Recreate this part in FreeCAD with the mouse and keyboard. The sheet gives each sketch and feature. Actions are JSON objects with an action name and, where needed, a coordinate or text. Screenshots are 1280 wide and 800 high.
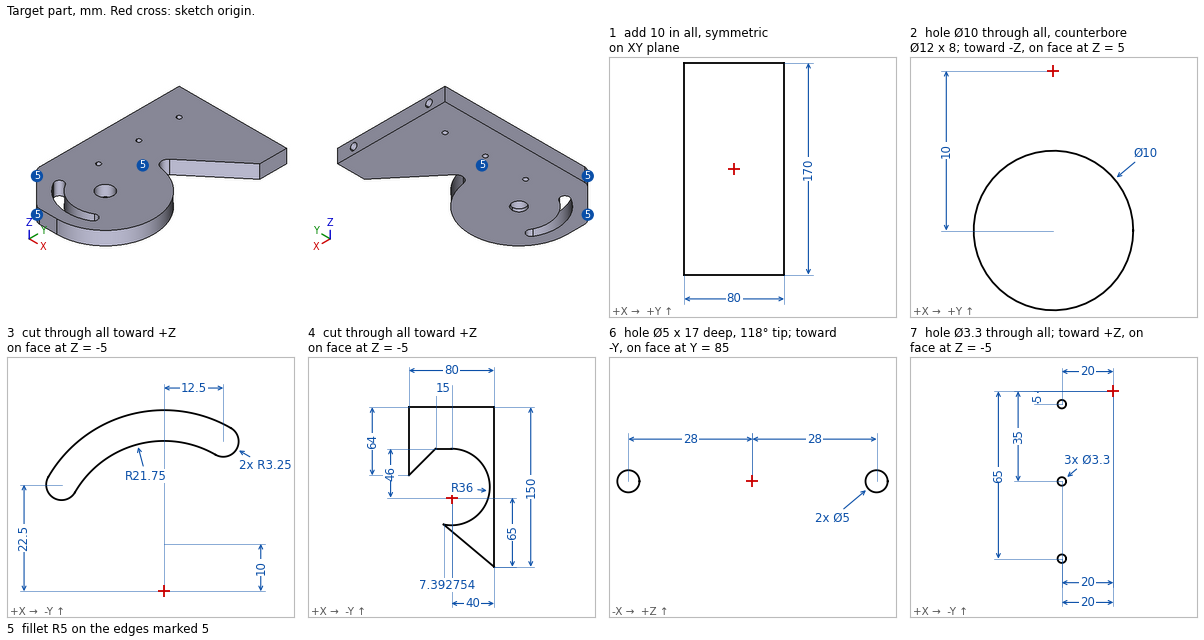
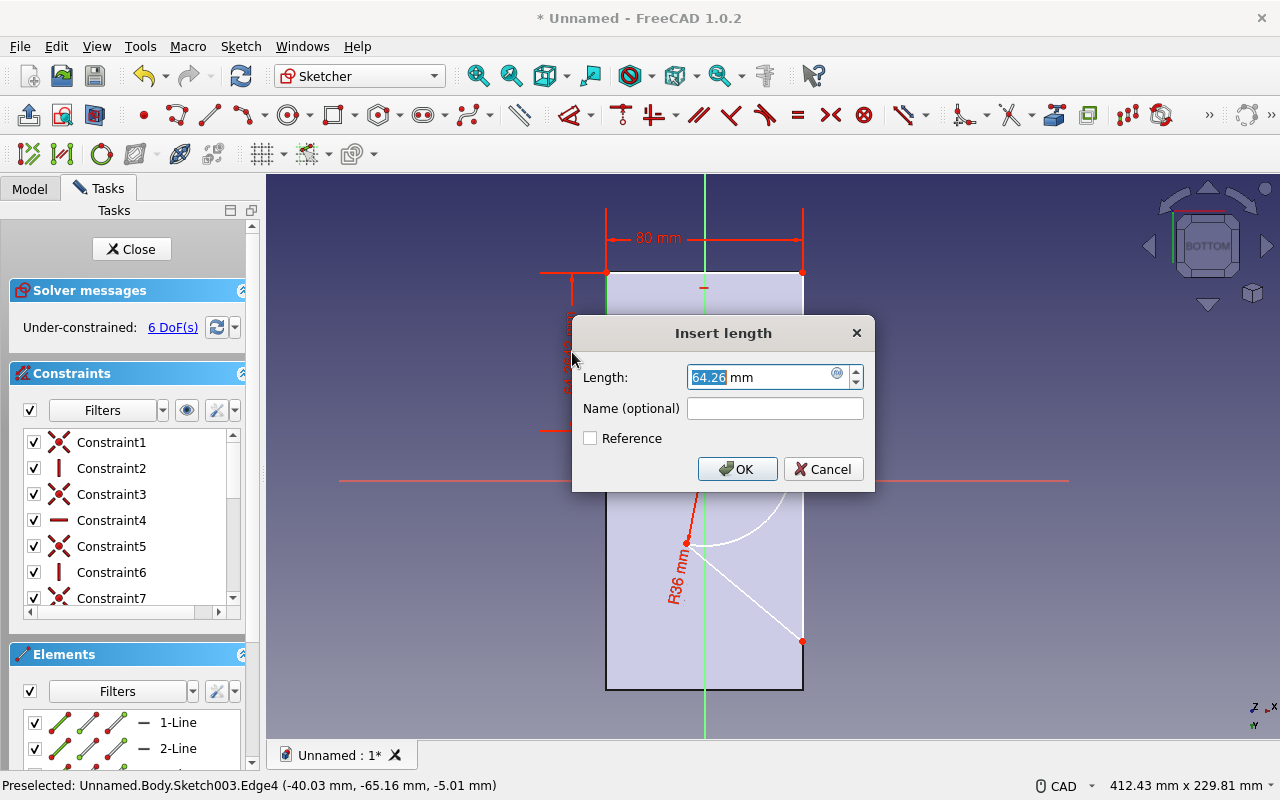
{"action": "type", "text": "64"}
{"action": "key", "text": "Return"}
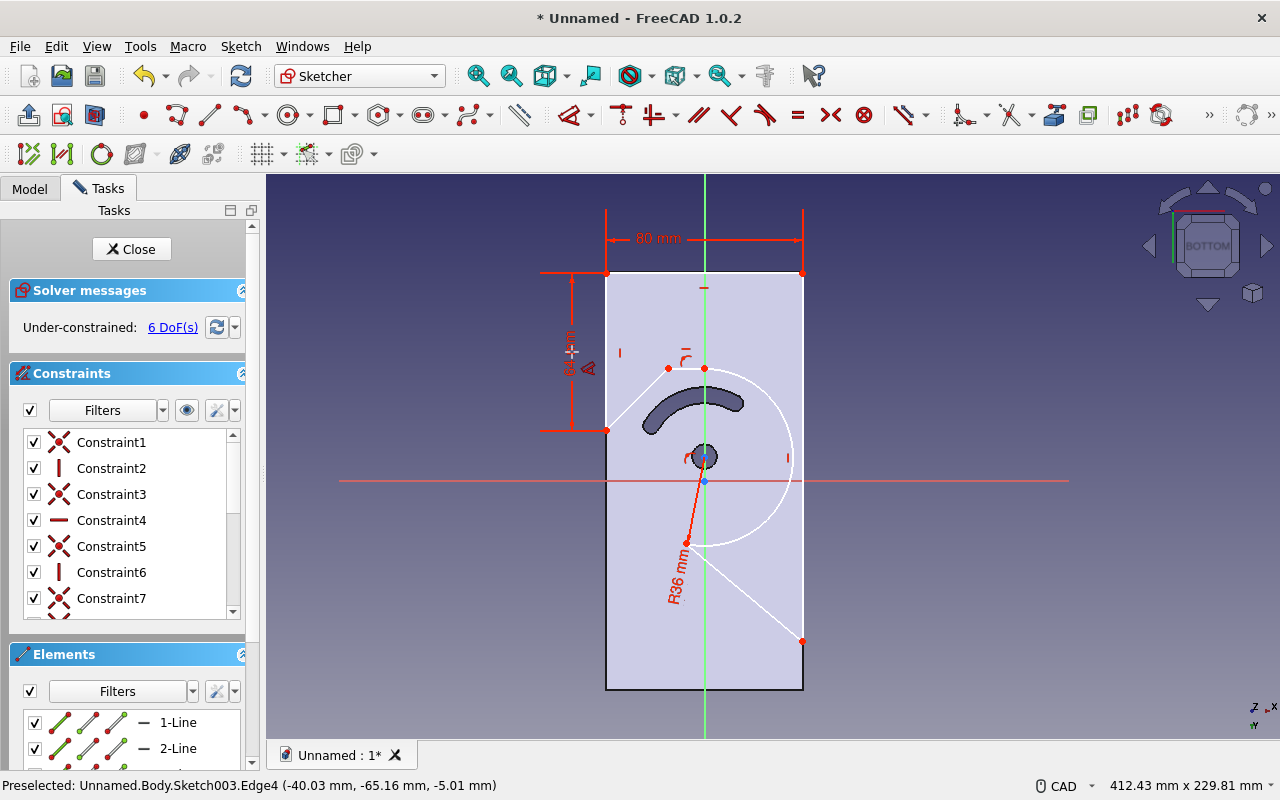
{"action": "scroll", "coordinate": [679, 369], "scroll_direction": "up", "scroll_amount": 2}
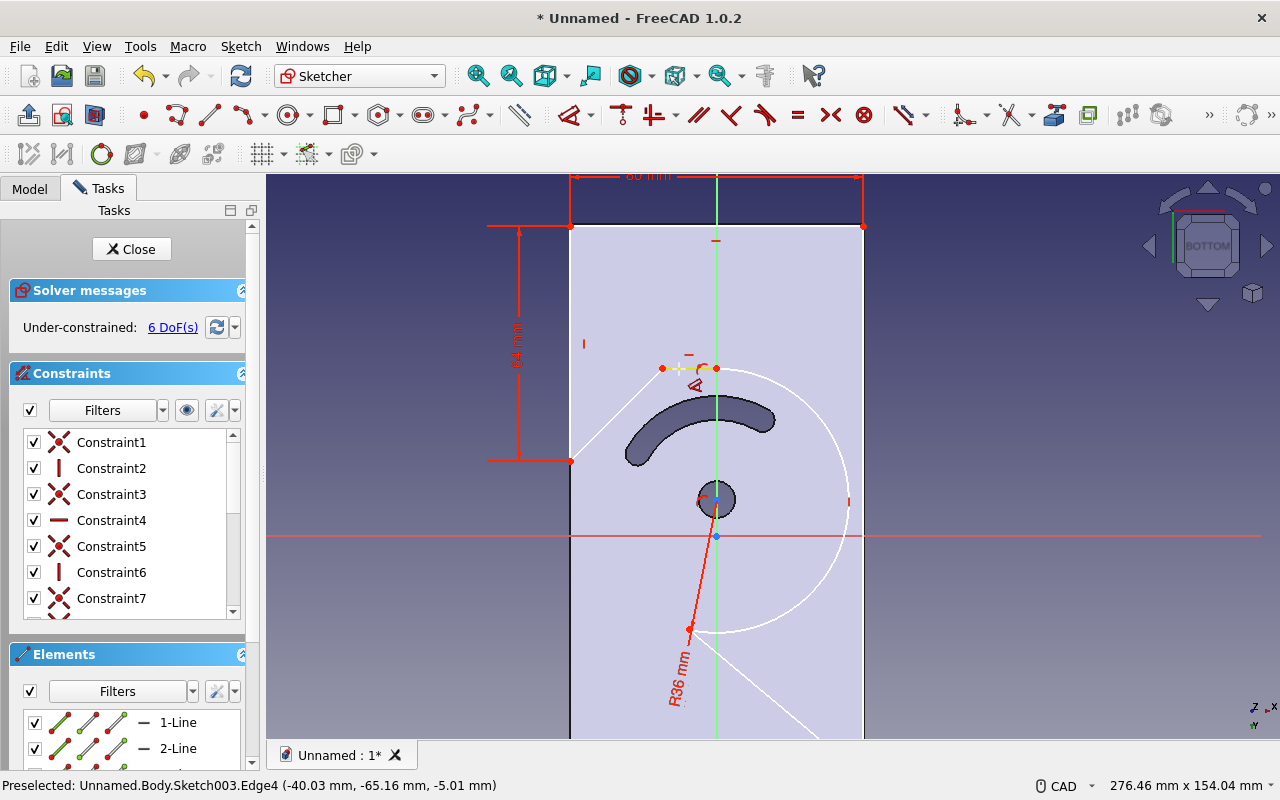
{"action": "left_click", "coordinate": [679, 369]}
{"action": "left_click", "coordinate": [690, 335]}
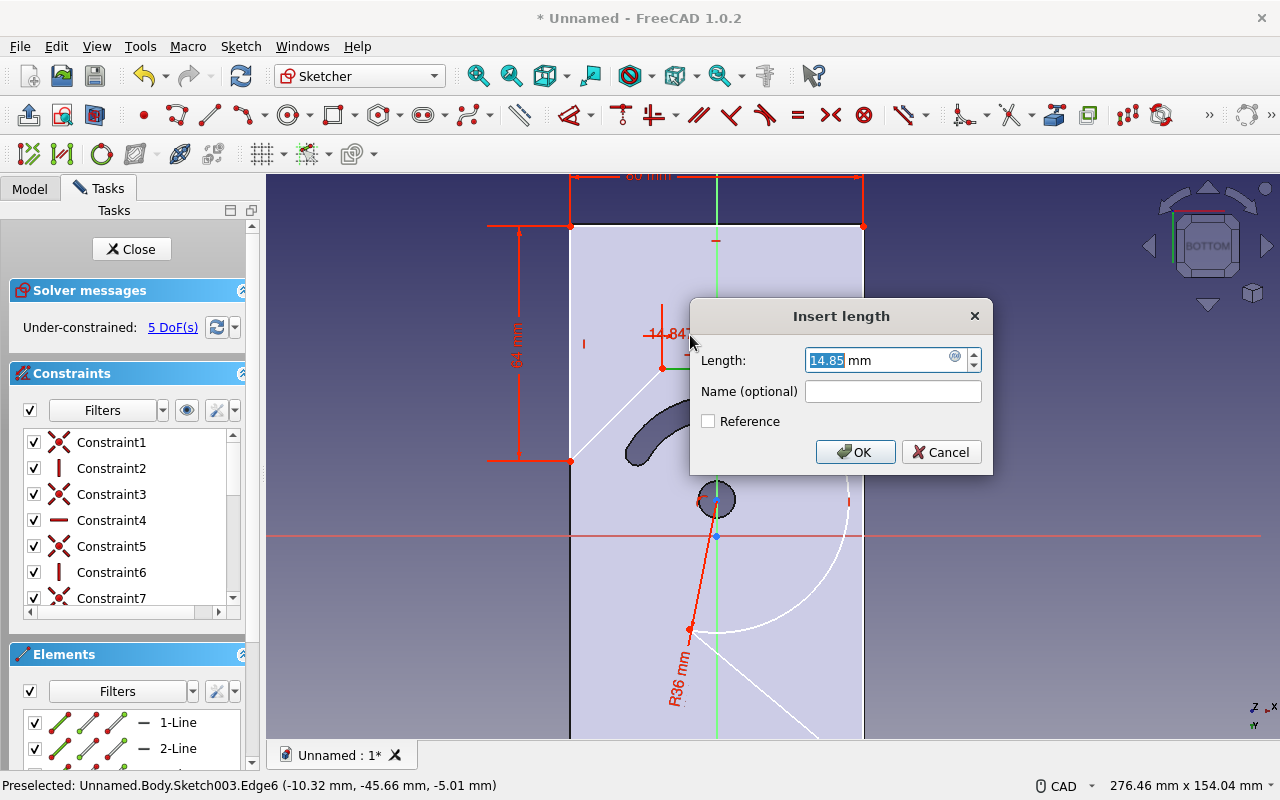
{"action": "type", "text": "15"}
{"action": "key", "text": "Return"}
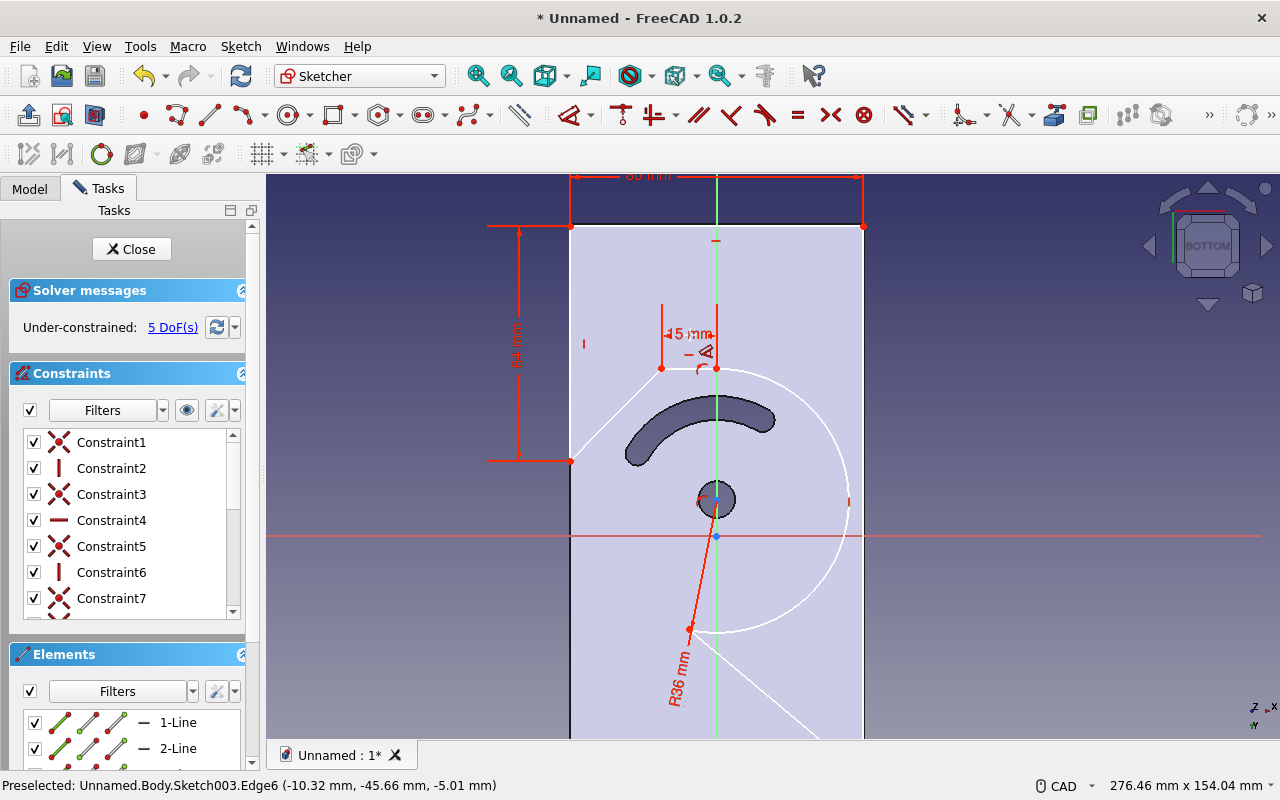
{"action": "left_click", "coordinate": [863, 611]}
{"action": "left_click", "coordinate": [897, 469]}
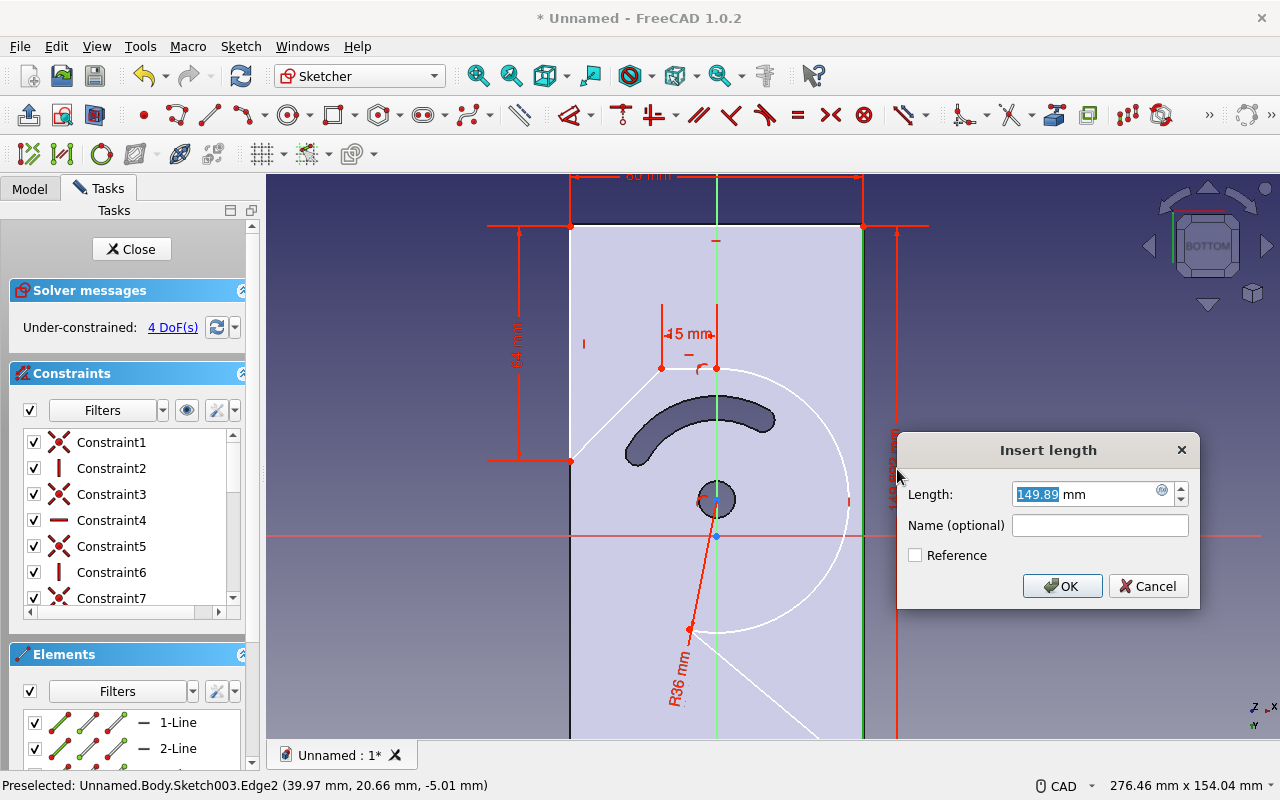
{"action": "type", "text": "150"}
{"action": "key", "text": "Return"}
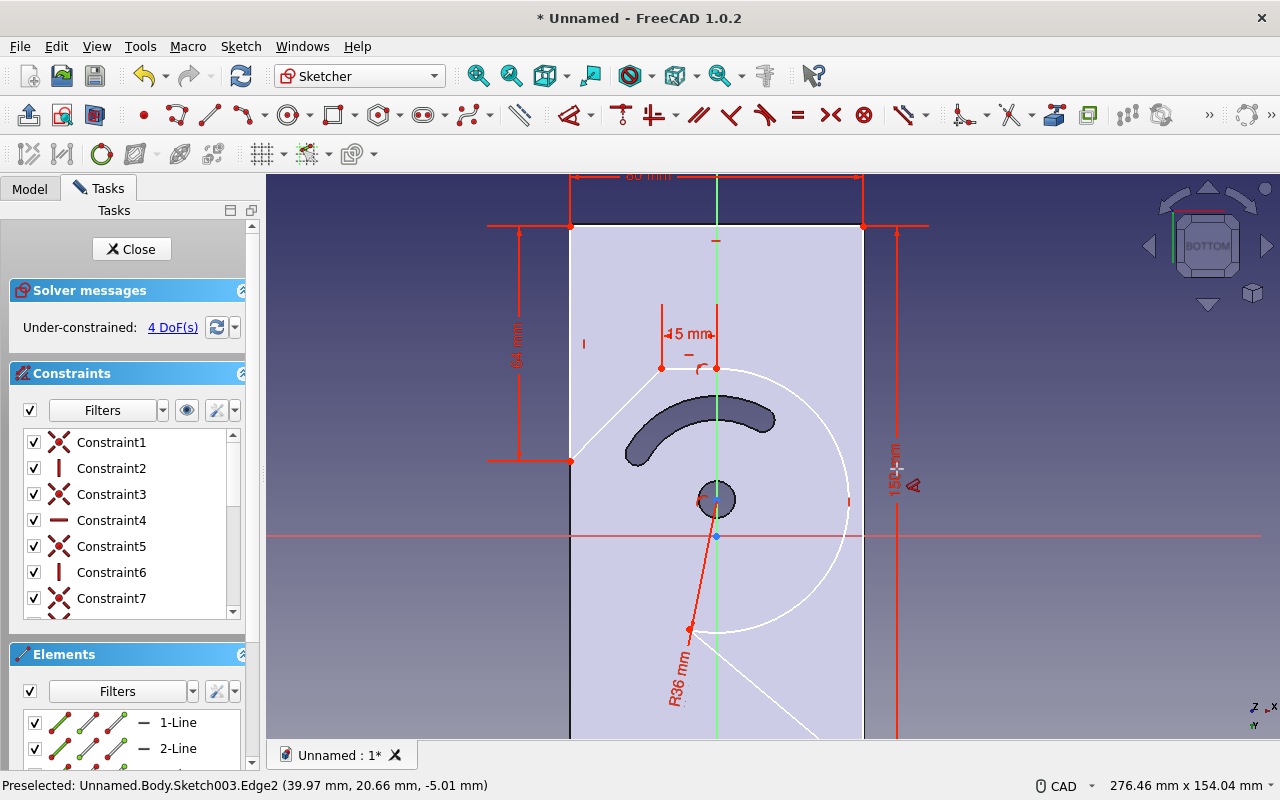
{"action": "scroll", "coordinate": [679, 369], "scroll_direction": "down", "scroll_amount": 2}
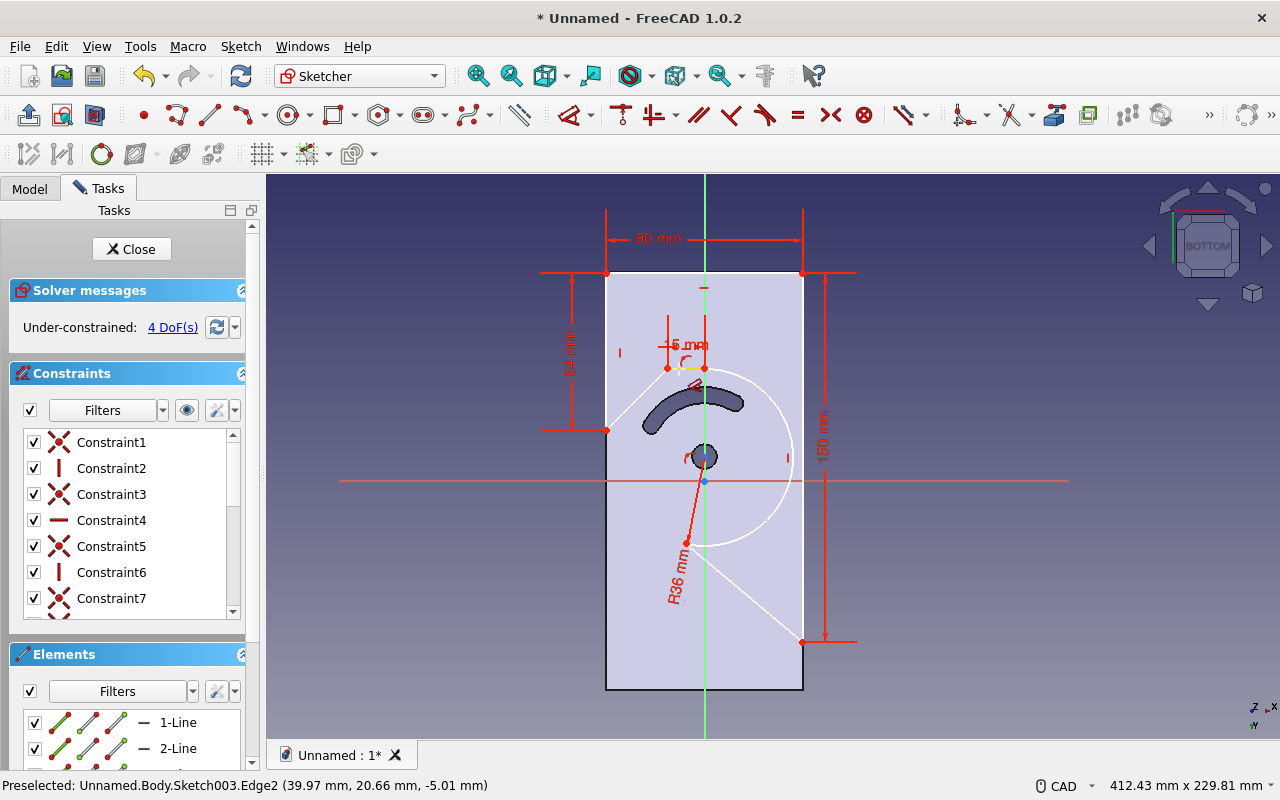
{"action": "left_click", "coordinate": [803, 642]}
{"action": "left_click", "coordinate": [754, 676]}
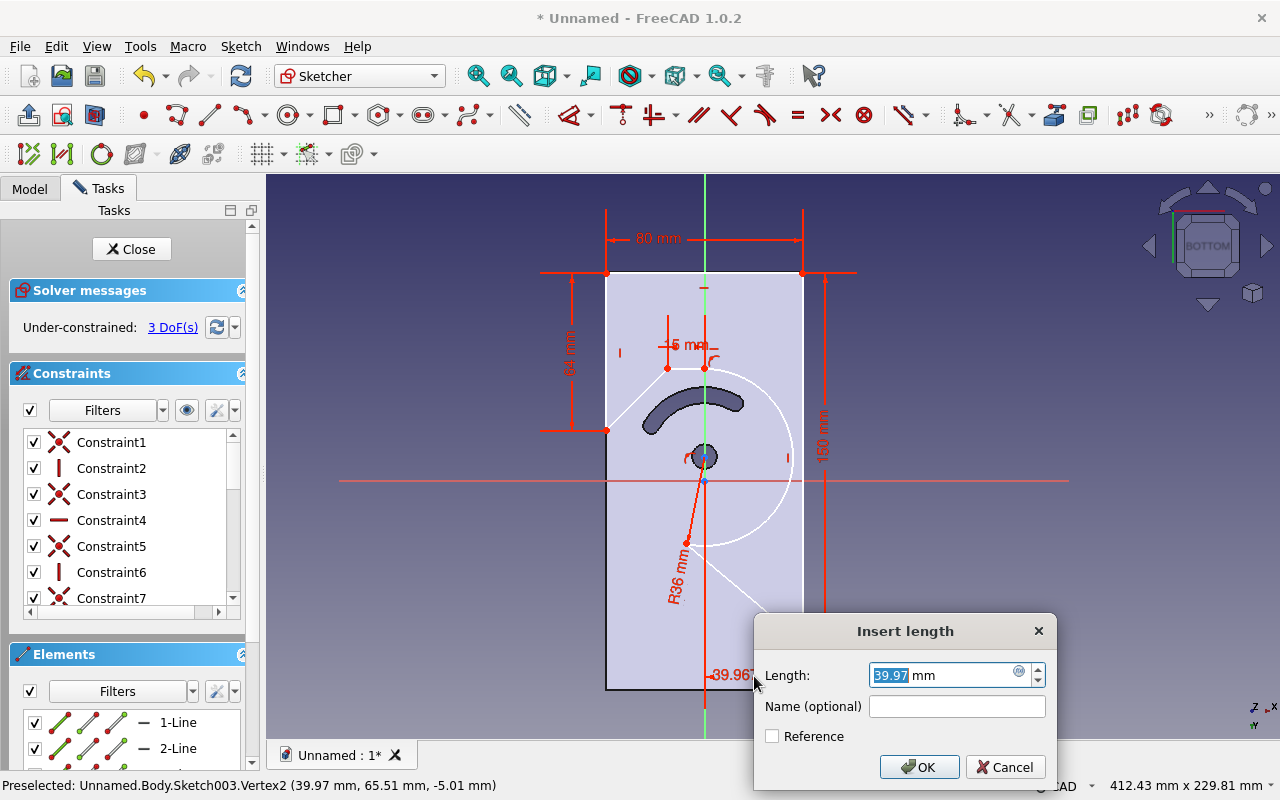
{"action": "type", "text": "40"}
{"action": "key", "text": "Return"}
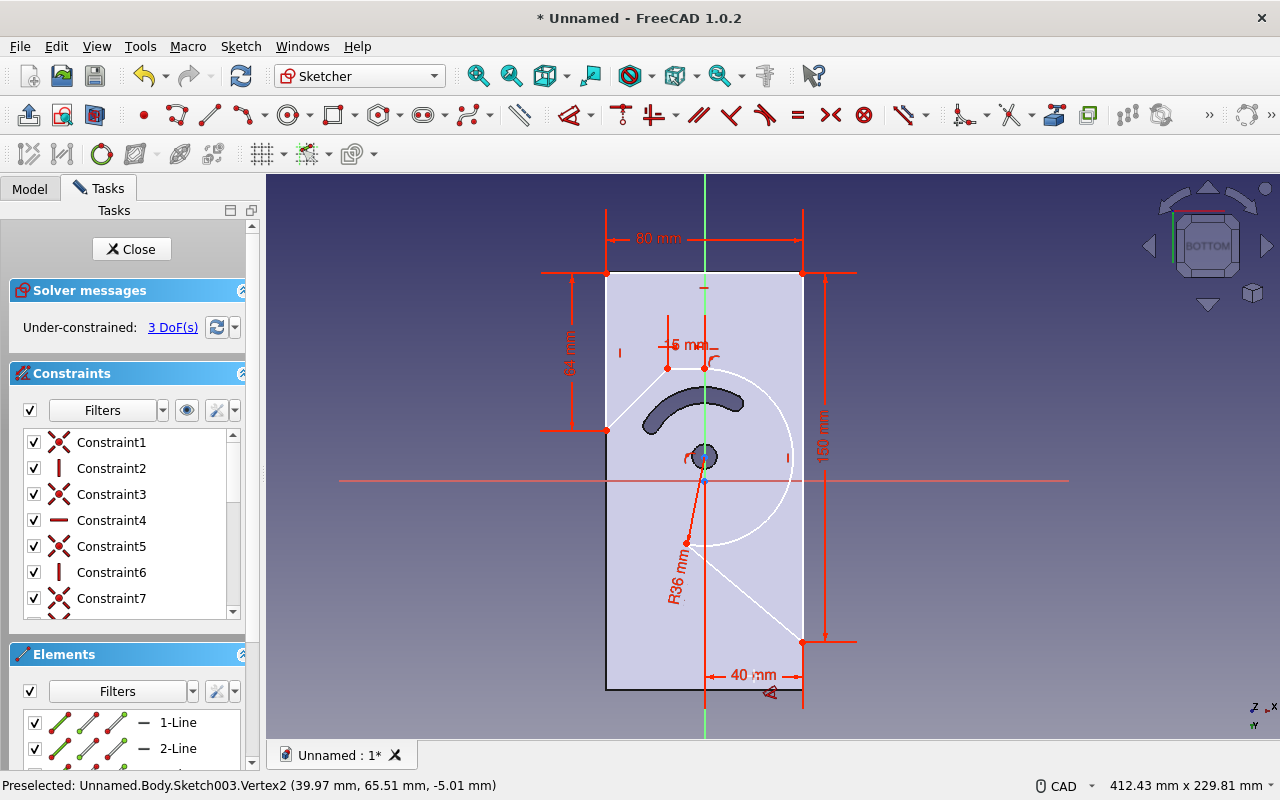
{"action": "left_click", "coordinate": [803, 642]}
{"action": "left_click", "coordinate": [837, 562]}